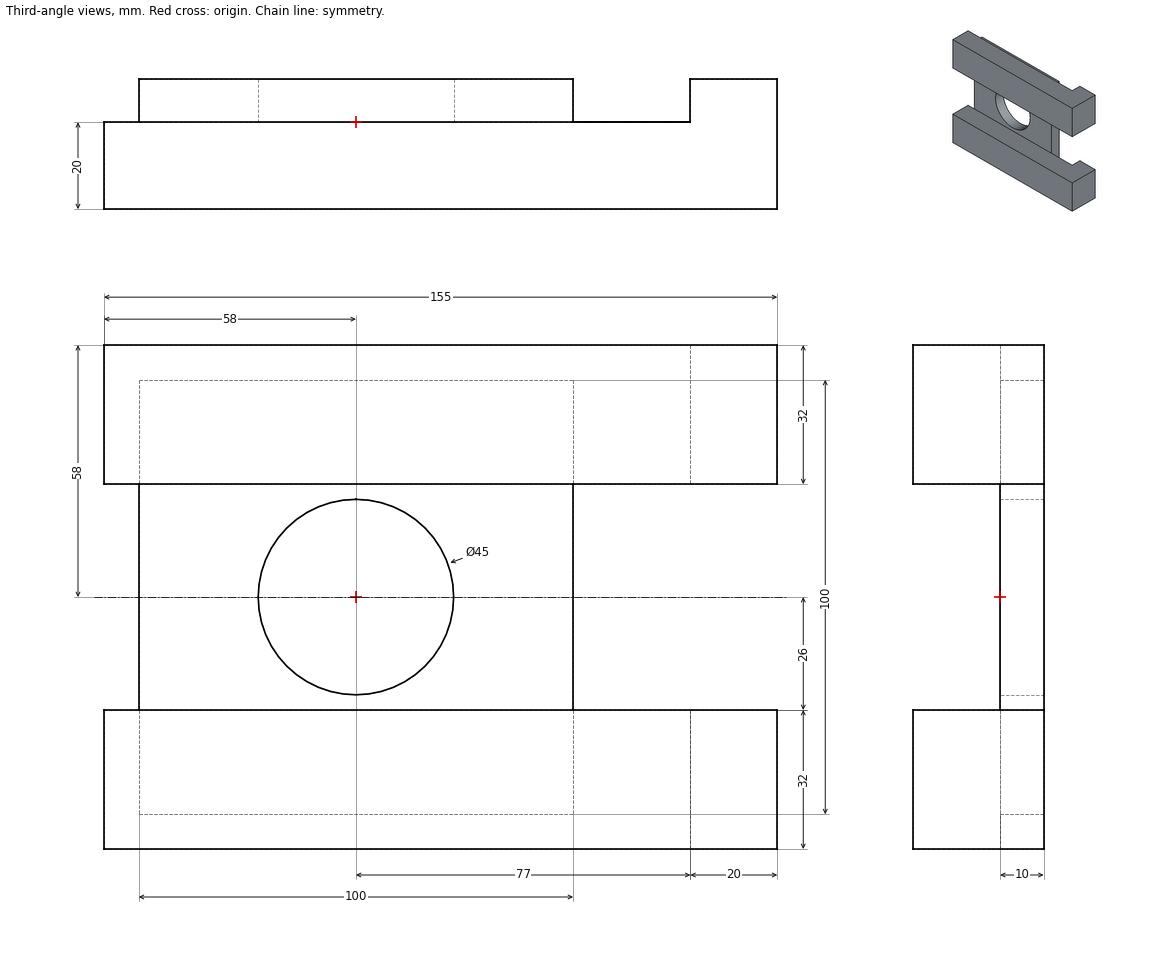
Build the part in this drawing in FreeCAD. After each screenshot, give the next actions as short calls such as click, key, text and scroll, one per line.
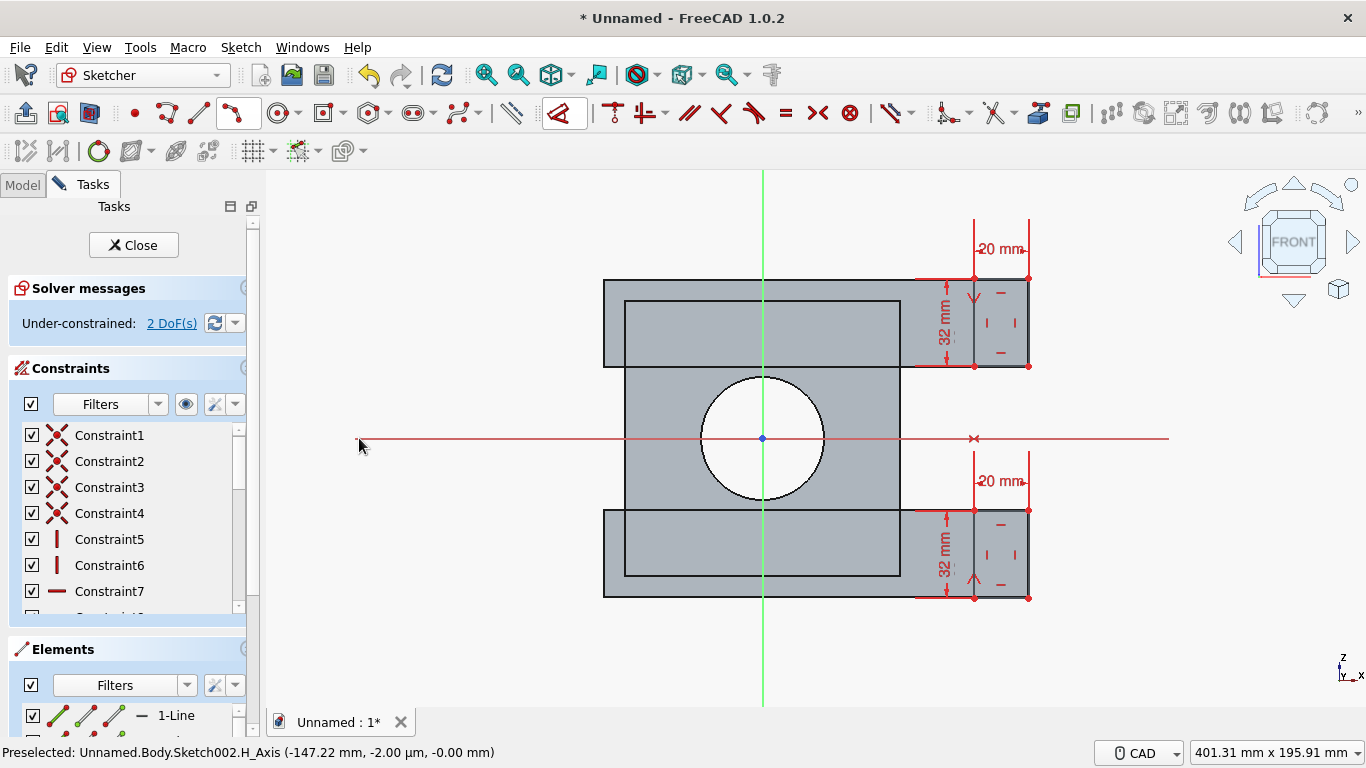
click(974, 511)
click(868, 545)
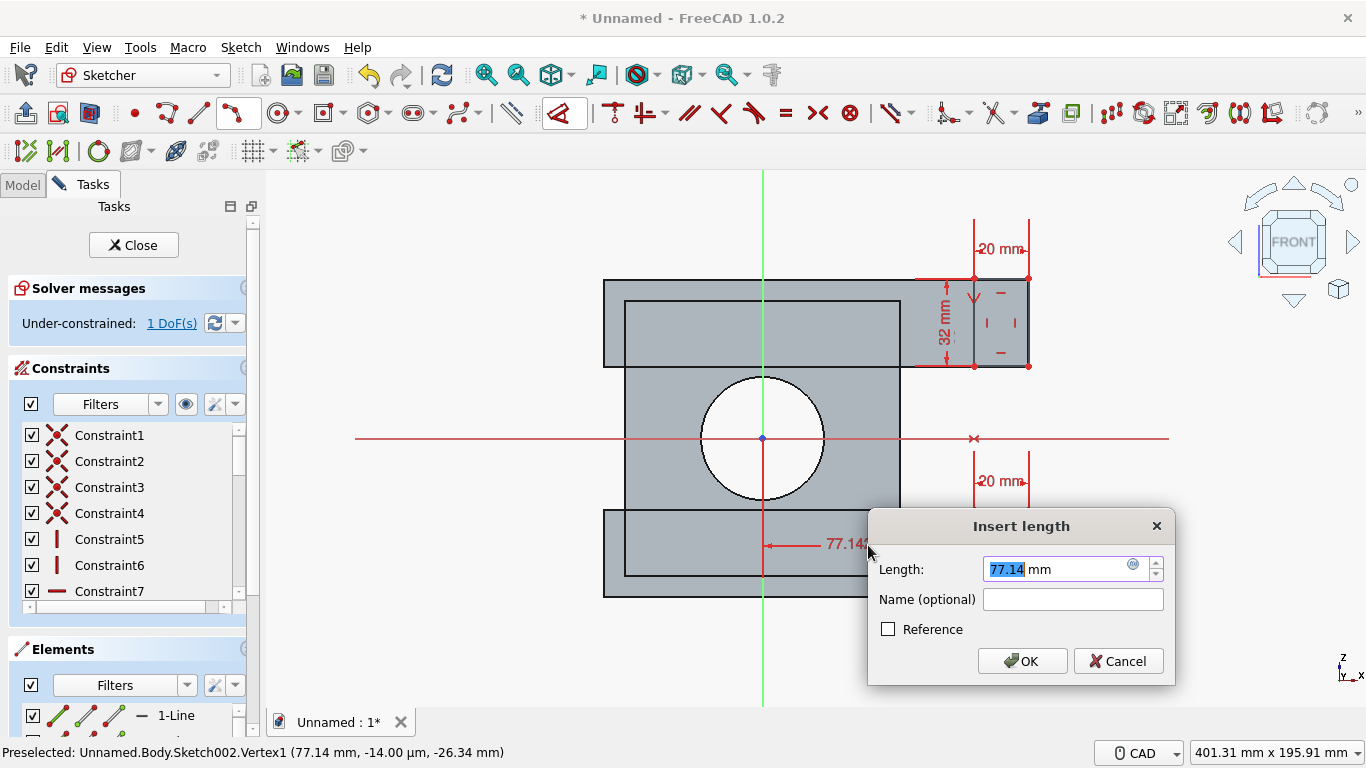
text(77)
key(Return)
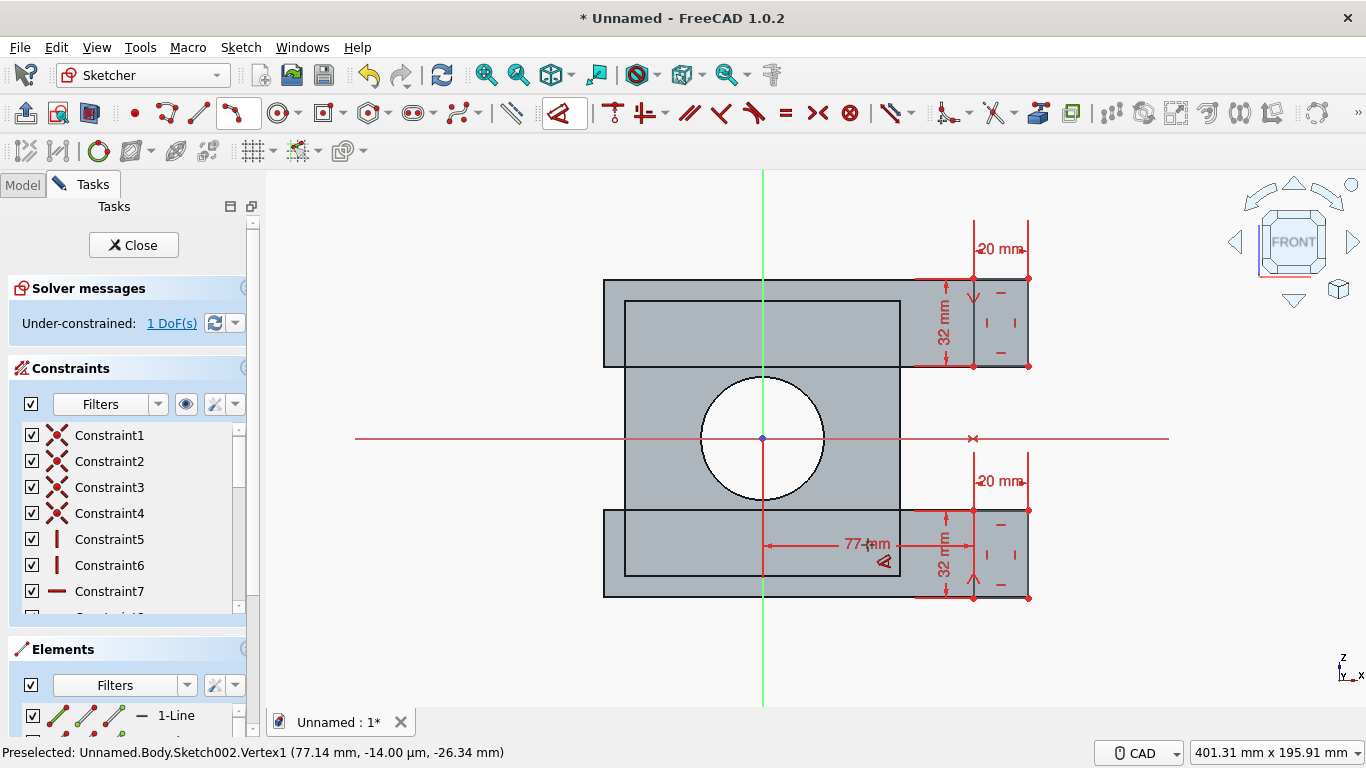
click(974, 511)
click(729, 475)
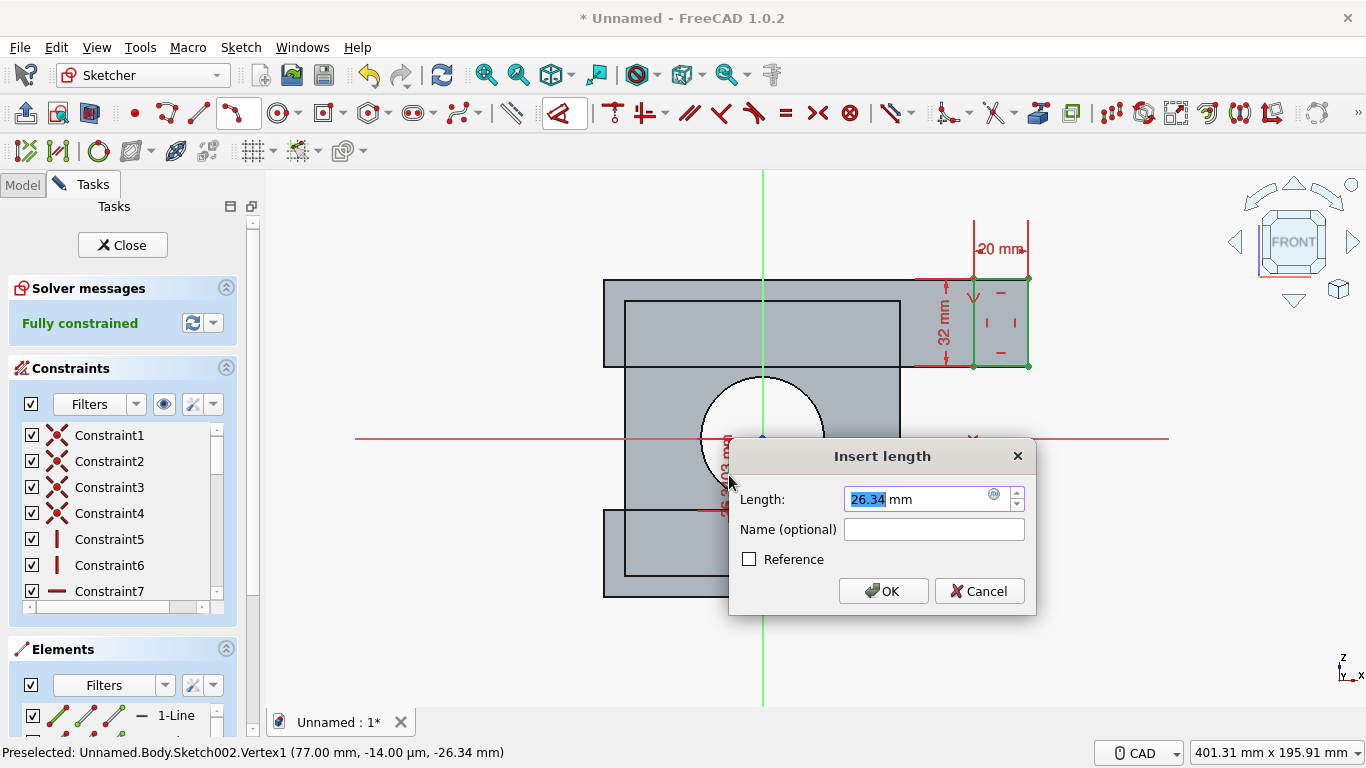
text(26)
key(Return)
key(Escape)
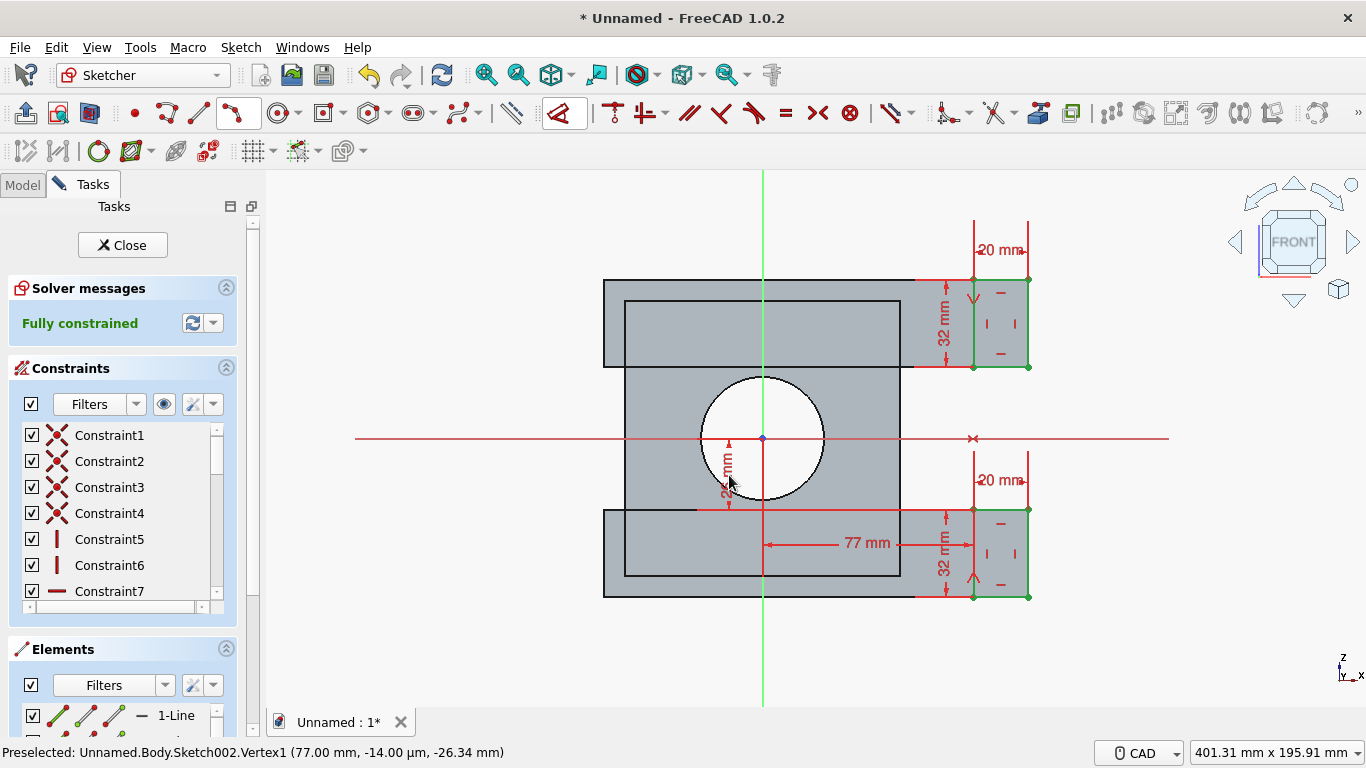
click(123, 245)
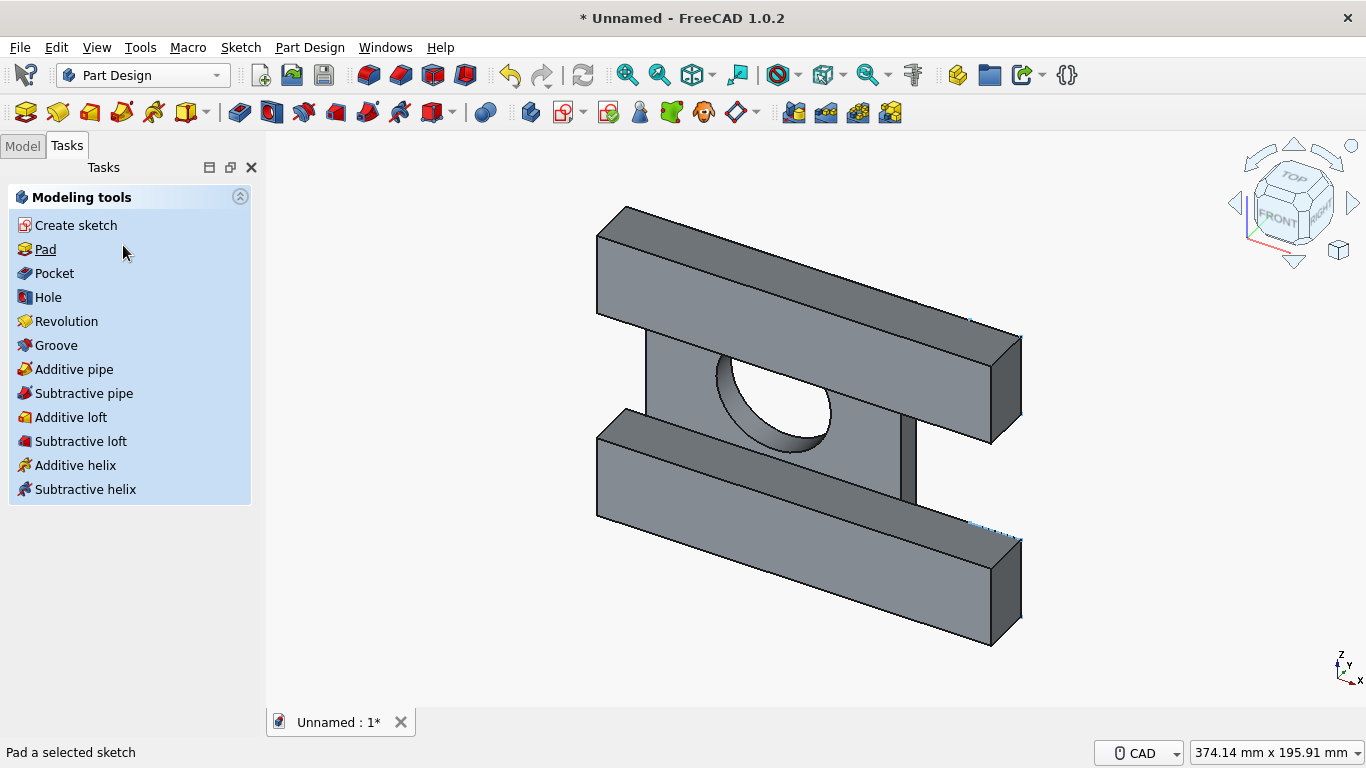
click(26, 112)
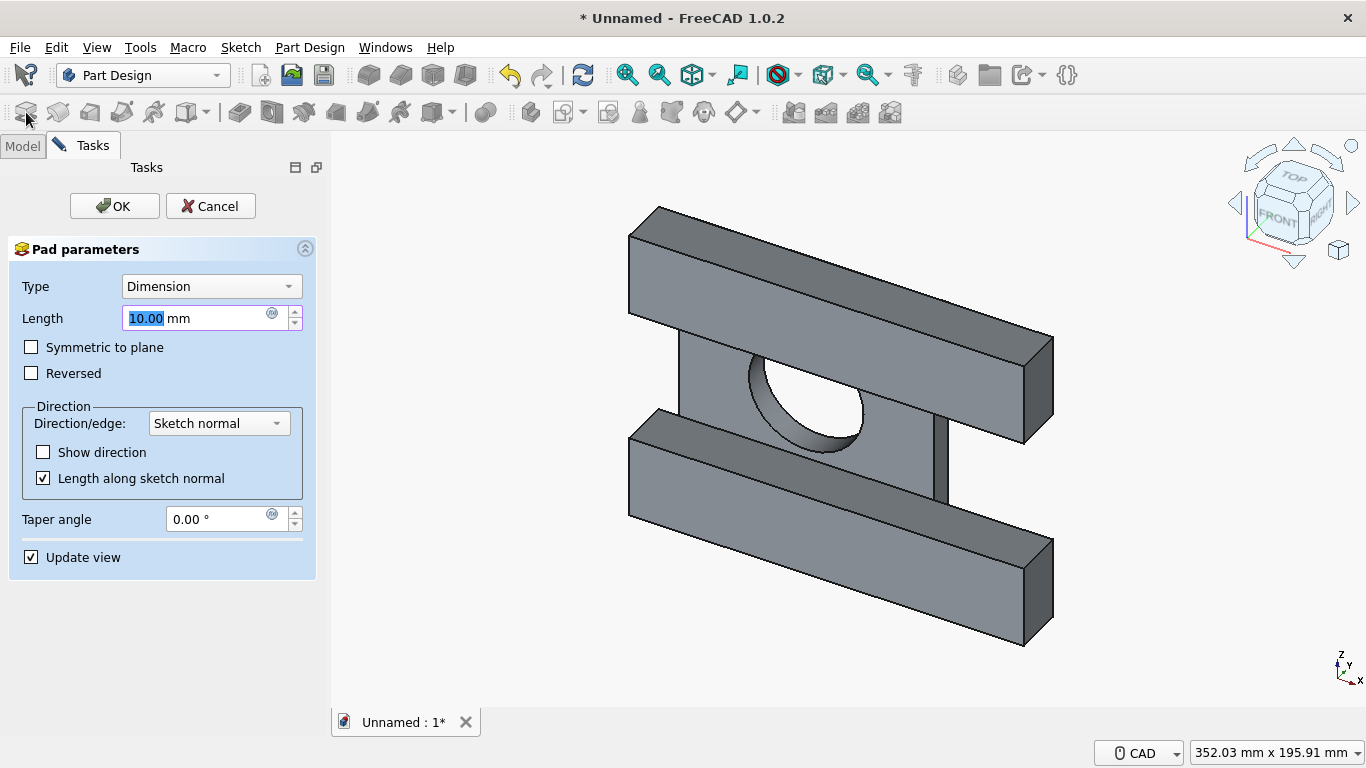
text(10)
key(Tab)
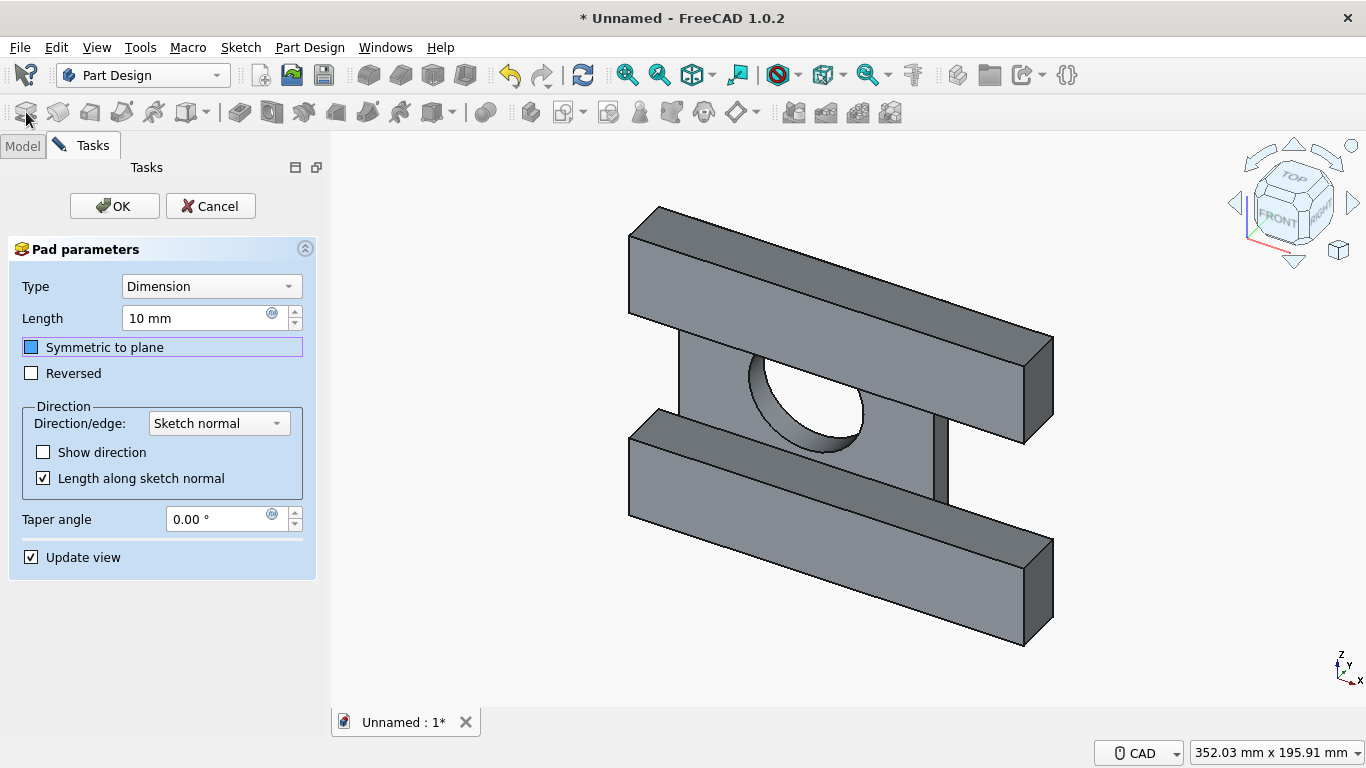
click(30, 373)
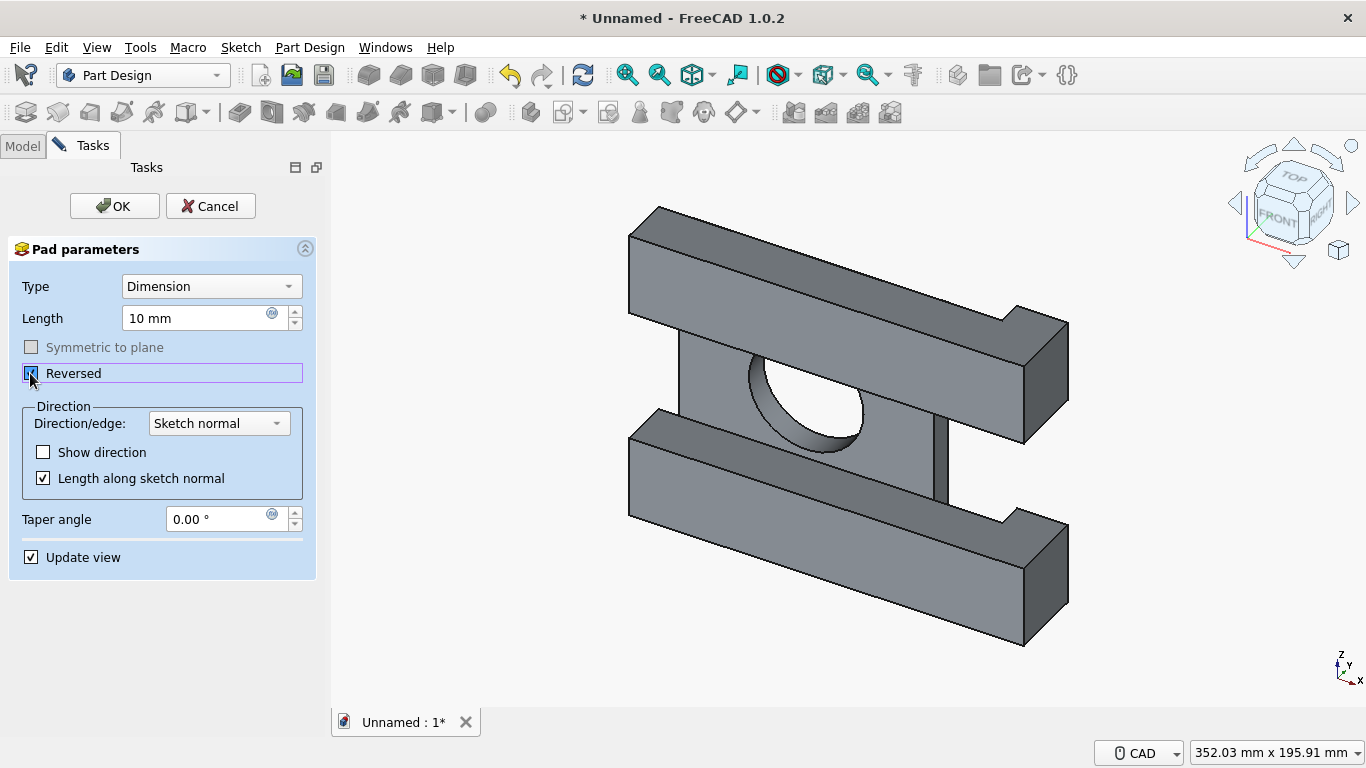
click(115, 206)